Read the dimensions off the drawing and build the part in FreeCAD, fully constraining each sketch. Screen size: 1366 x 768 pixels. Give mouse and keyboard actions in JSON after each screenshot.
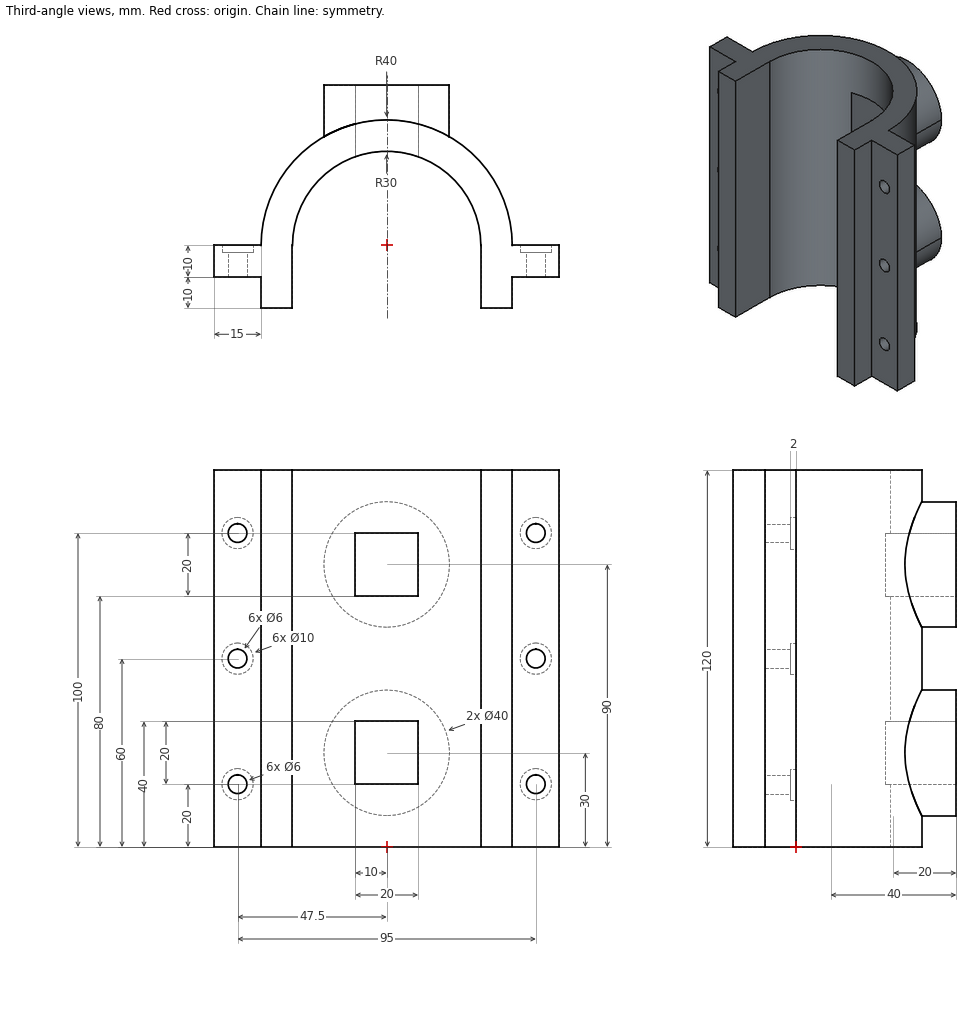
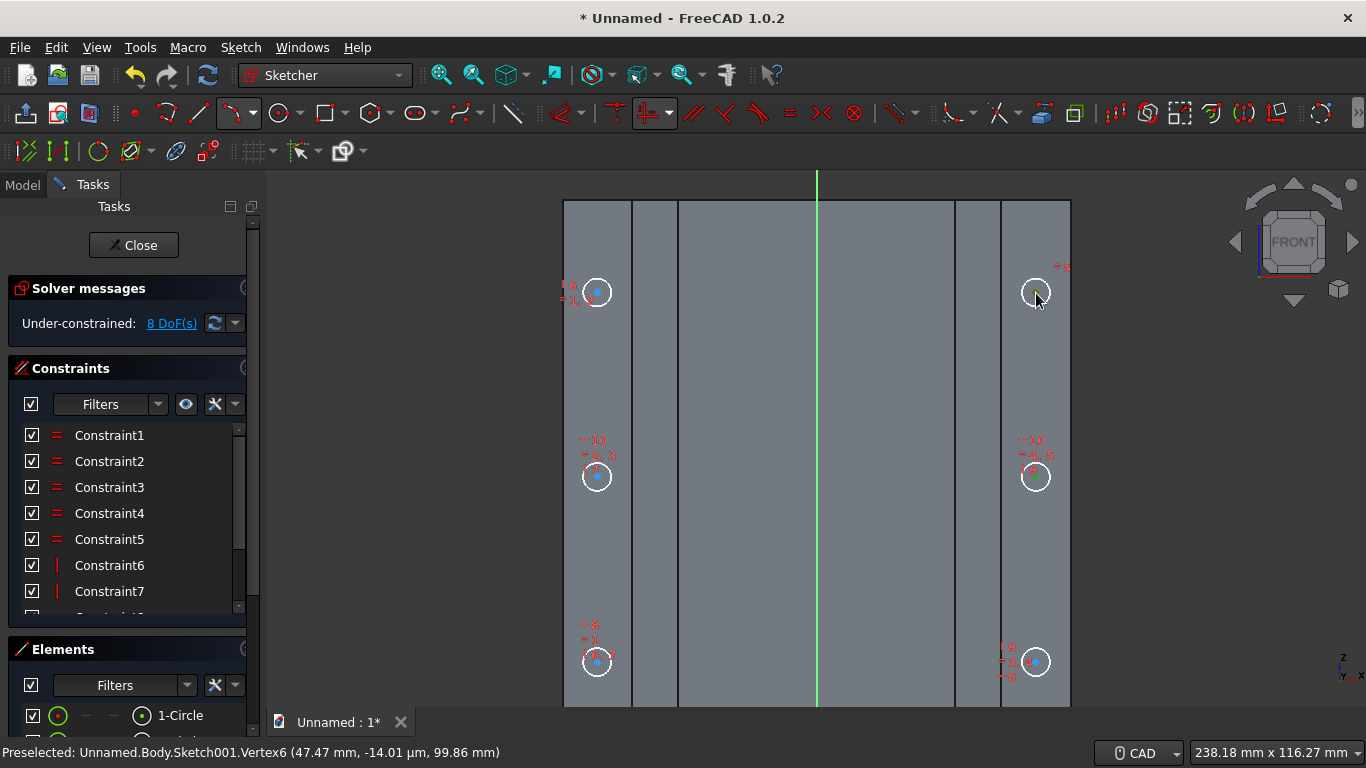
{"action": "left_click", "coordinate": [672, 114]}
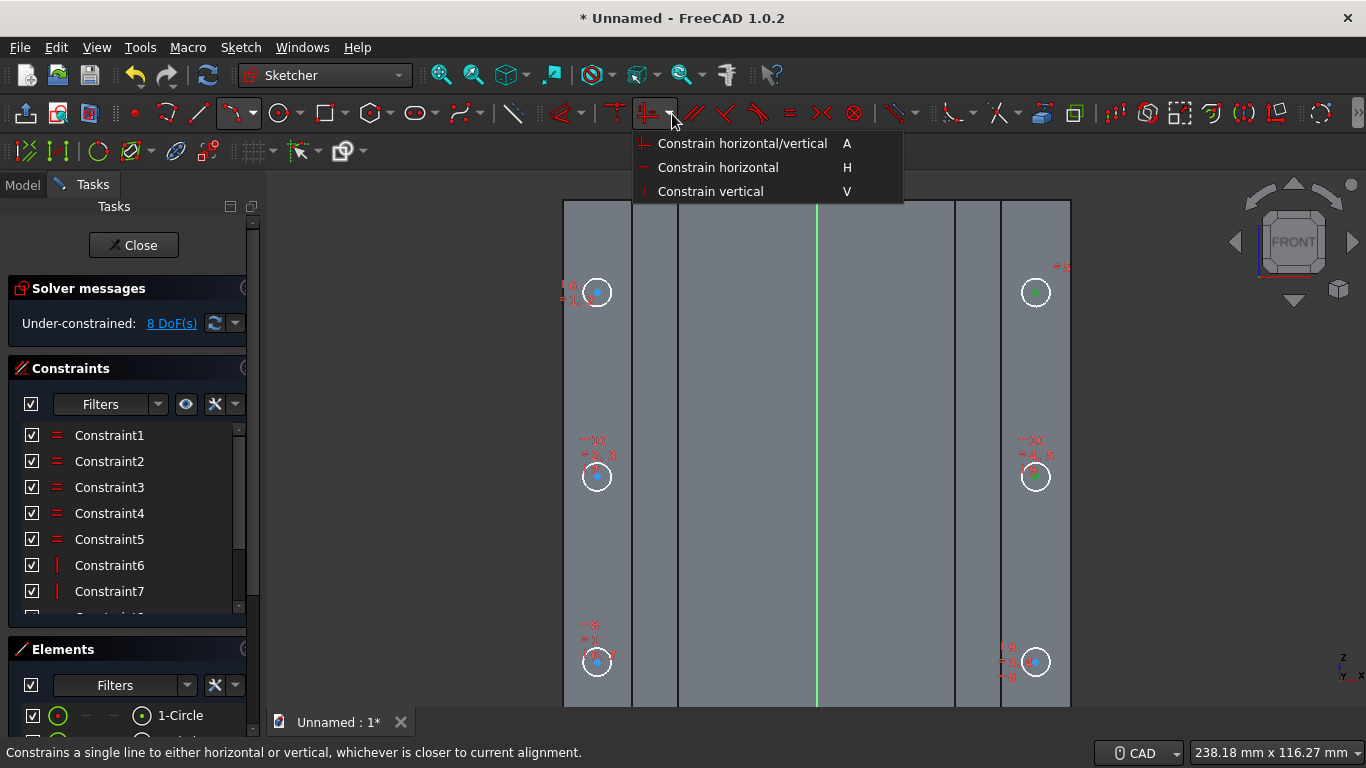
{"action": "left_click", "coordinate": [768, 191]}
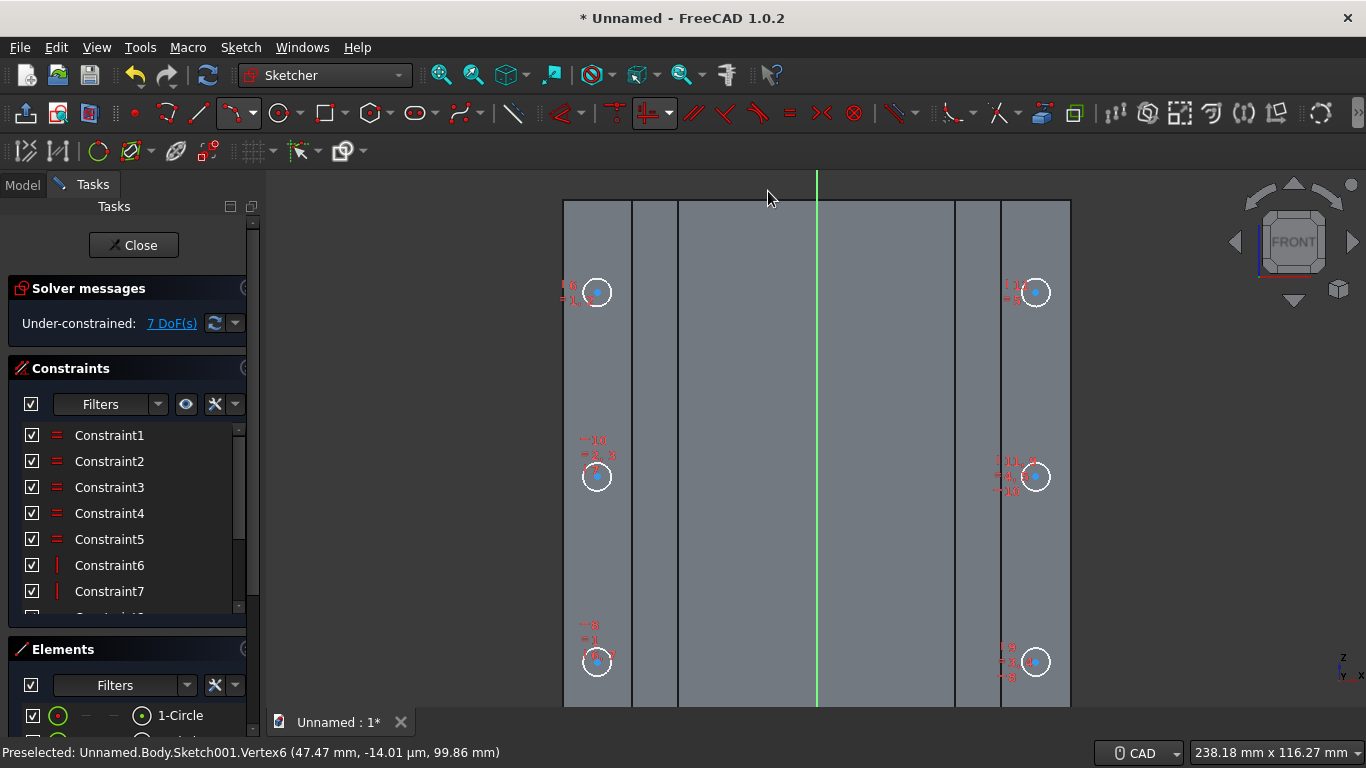
{"action": "left_click", "coordinate": [597, 293]}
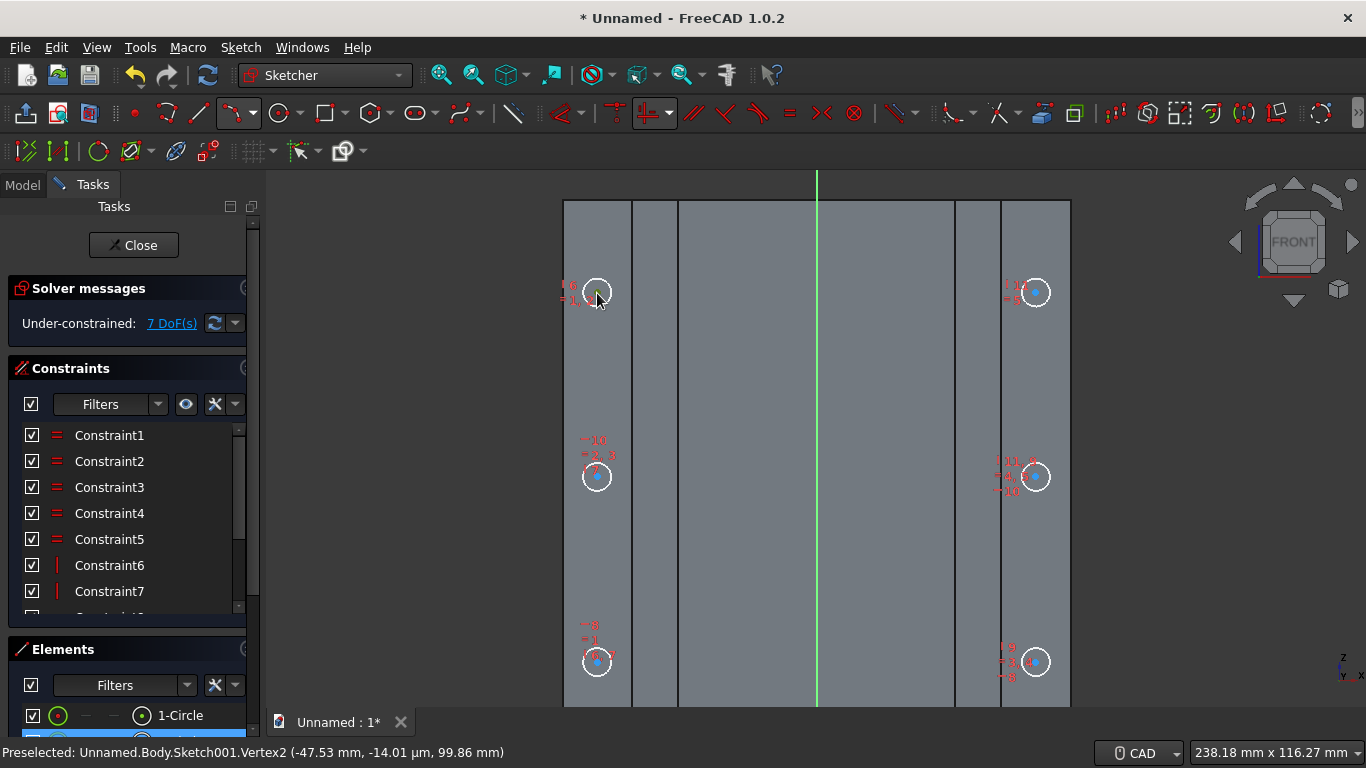
{"action": "left_click", "coordinate": [1036, 293]}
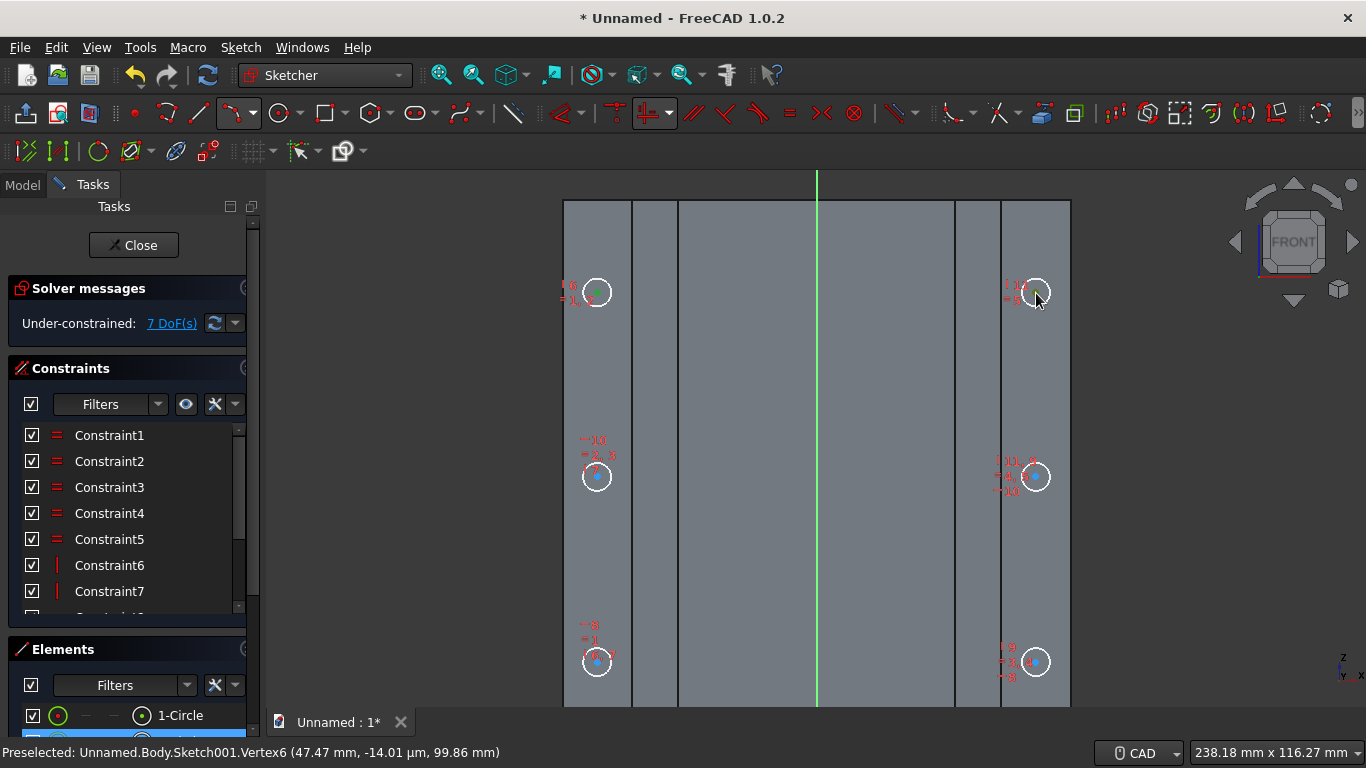
{"action": "left_click", "coordinate": [672, 114]}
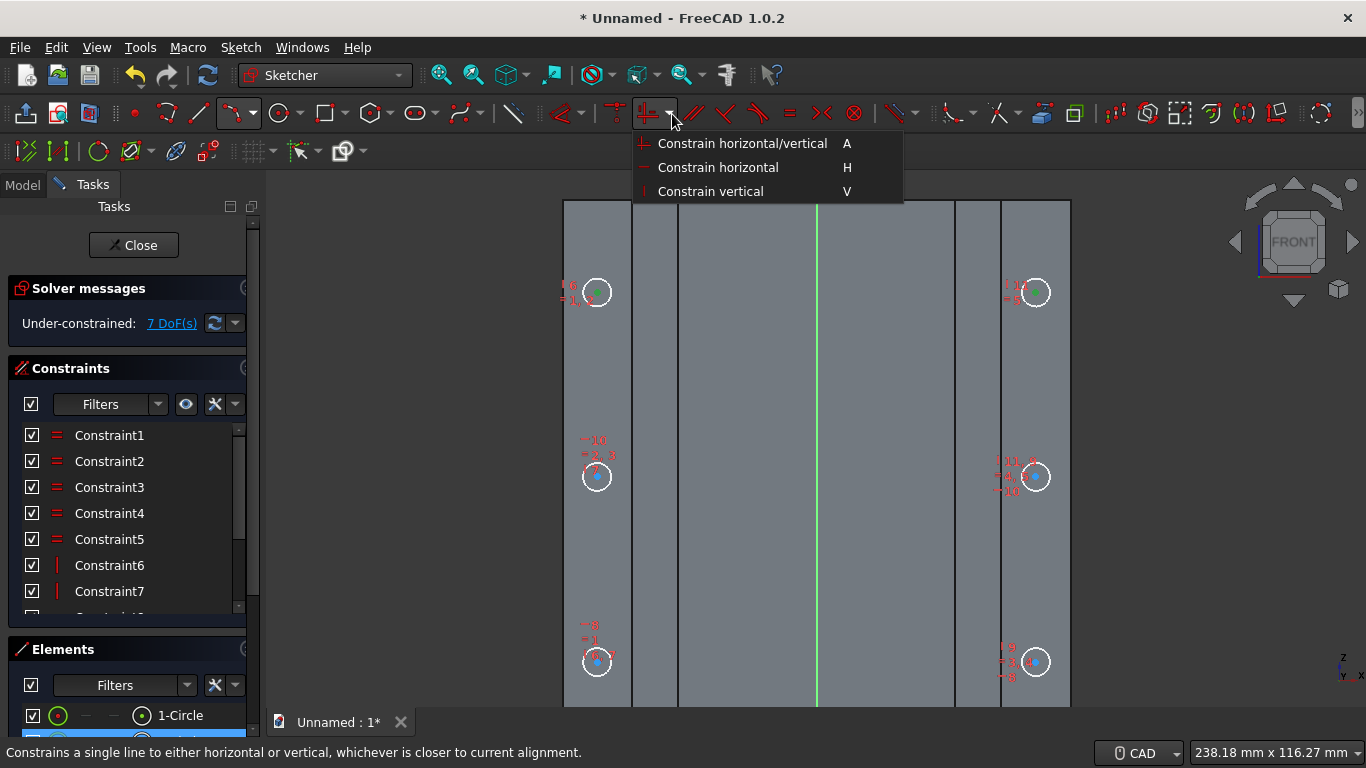
{"action": "left_click", "coordinate": [768, 167]}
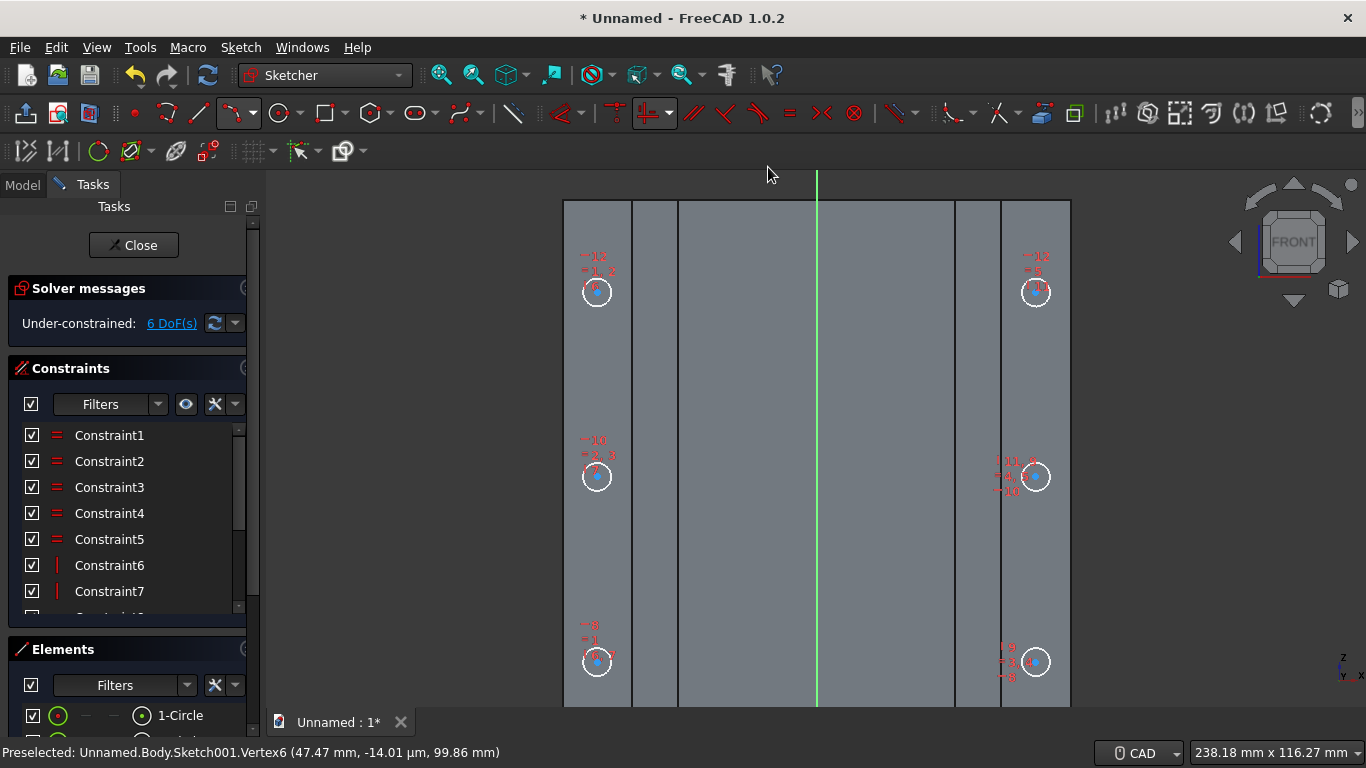
{"action": "left_click", "coordinate": [560, 114]}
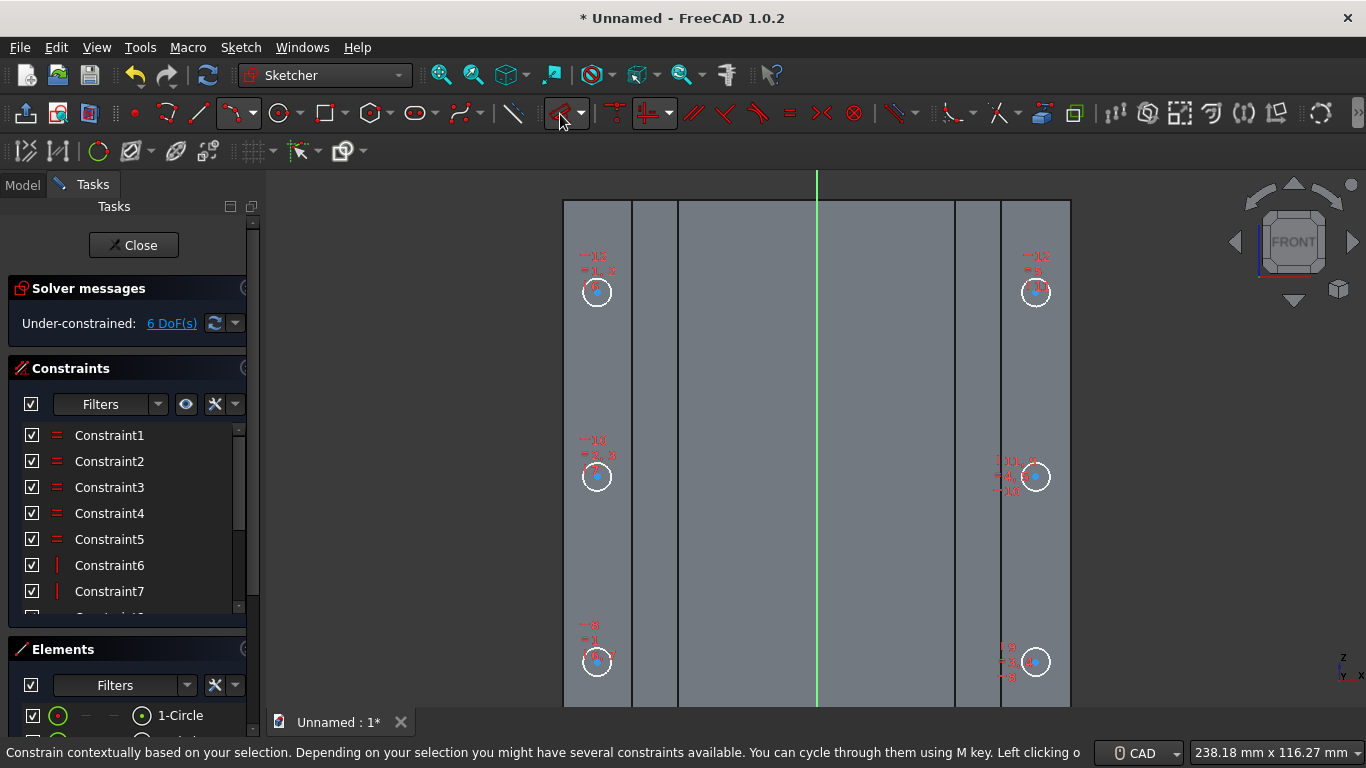
{"action": "scroll", "coordinate": [607, 652], "scroll_direction": "up", "scroll_amount": 2}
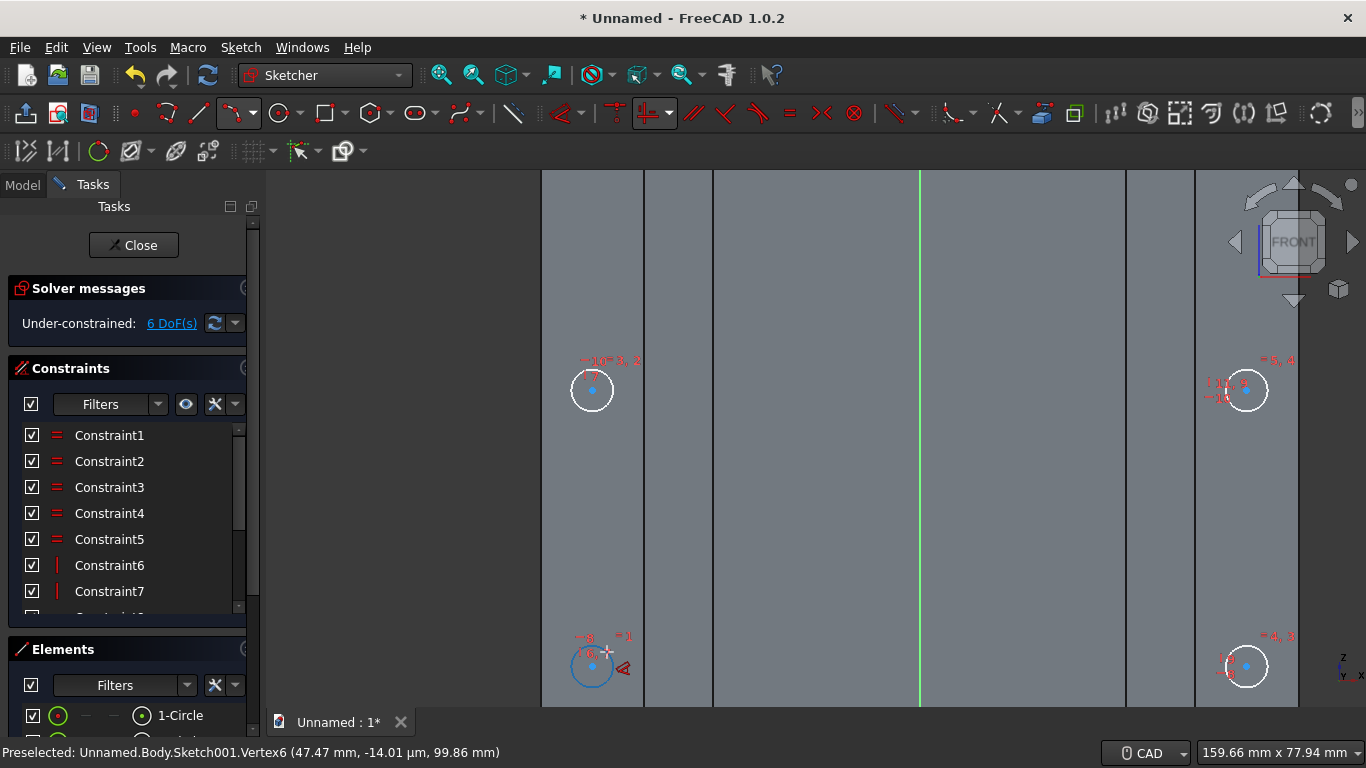
{"action": "left_click", "coordinate": [607, 652]}
{"action": "left_click", "coordinate": [630, 629]}